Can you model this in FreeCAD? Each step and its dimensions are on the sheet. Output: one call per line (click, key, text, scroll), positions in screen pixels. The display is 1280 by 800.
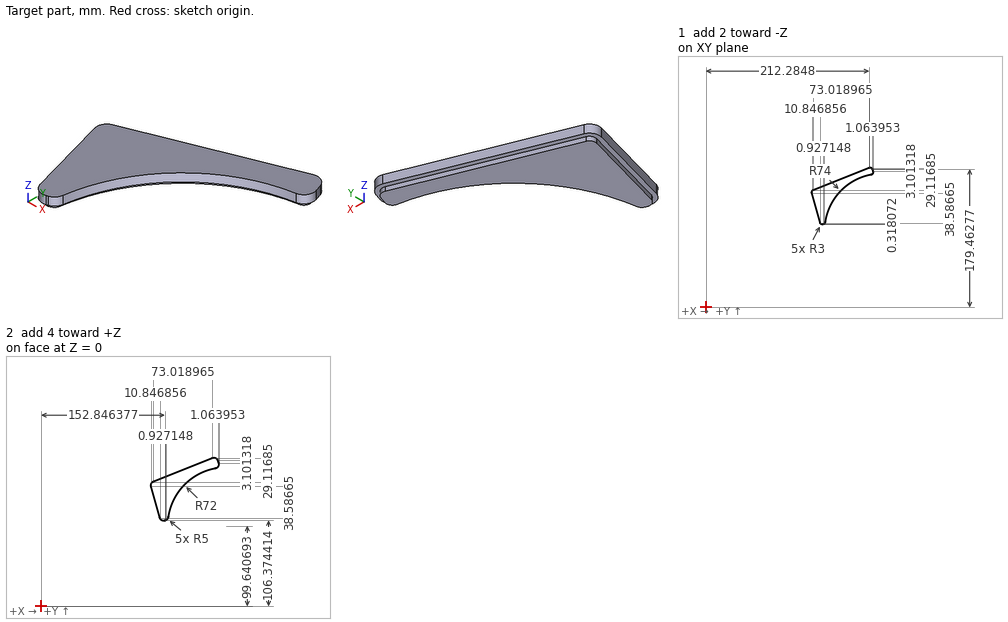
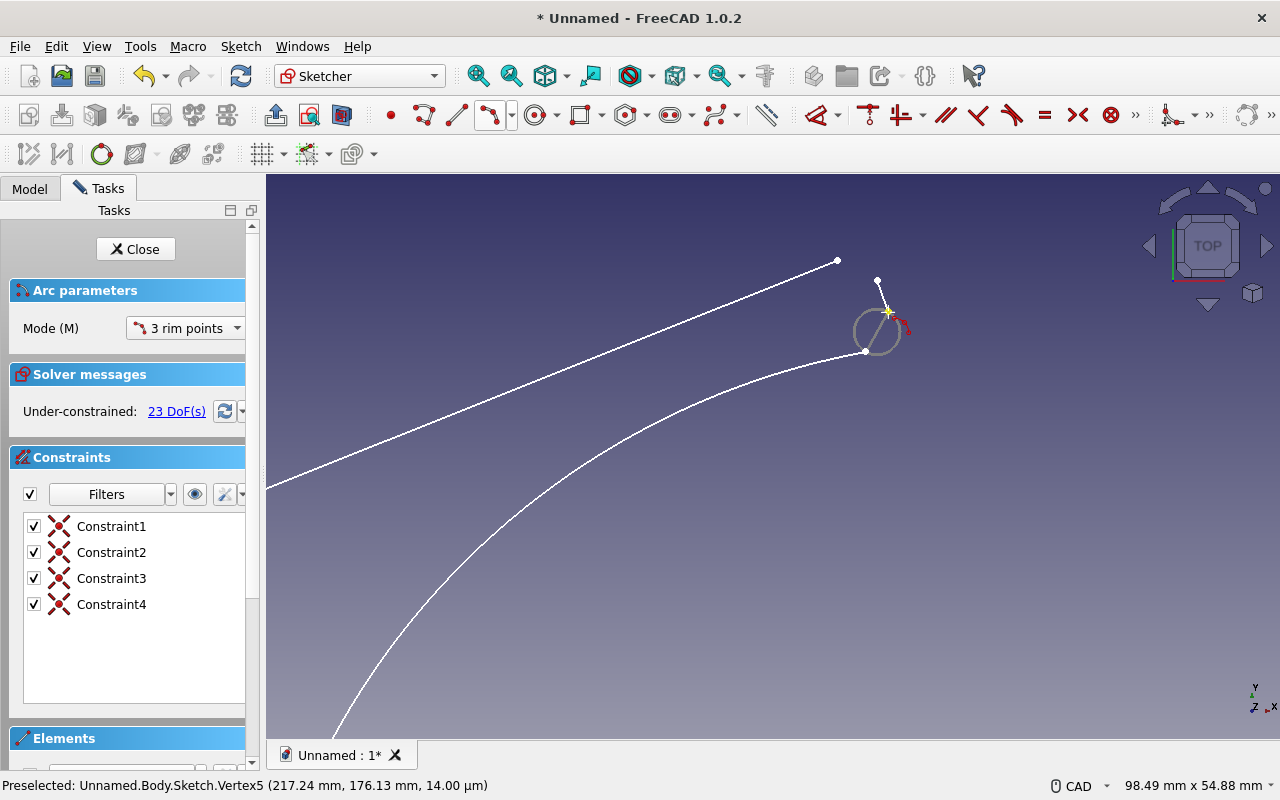
scroll(886, 335, up, 2)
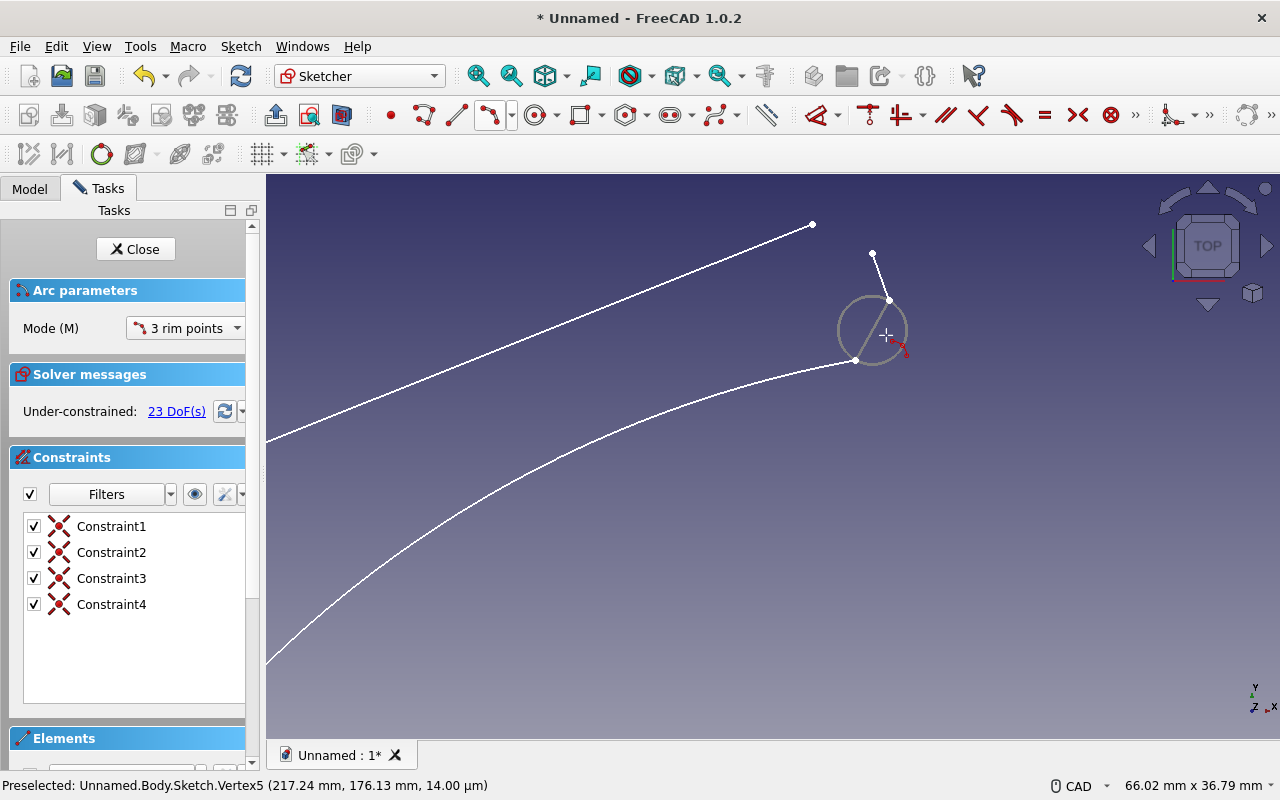
click(886, 335)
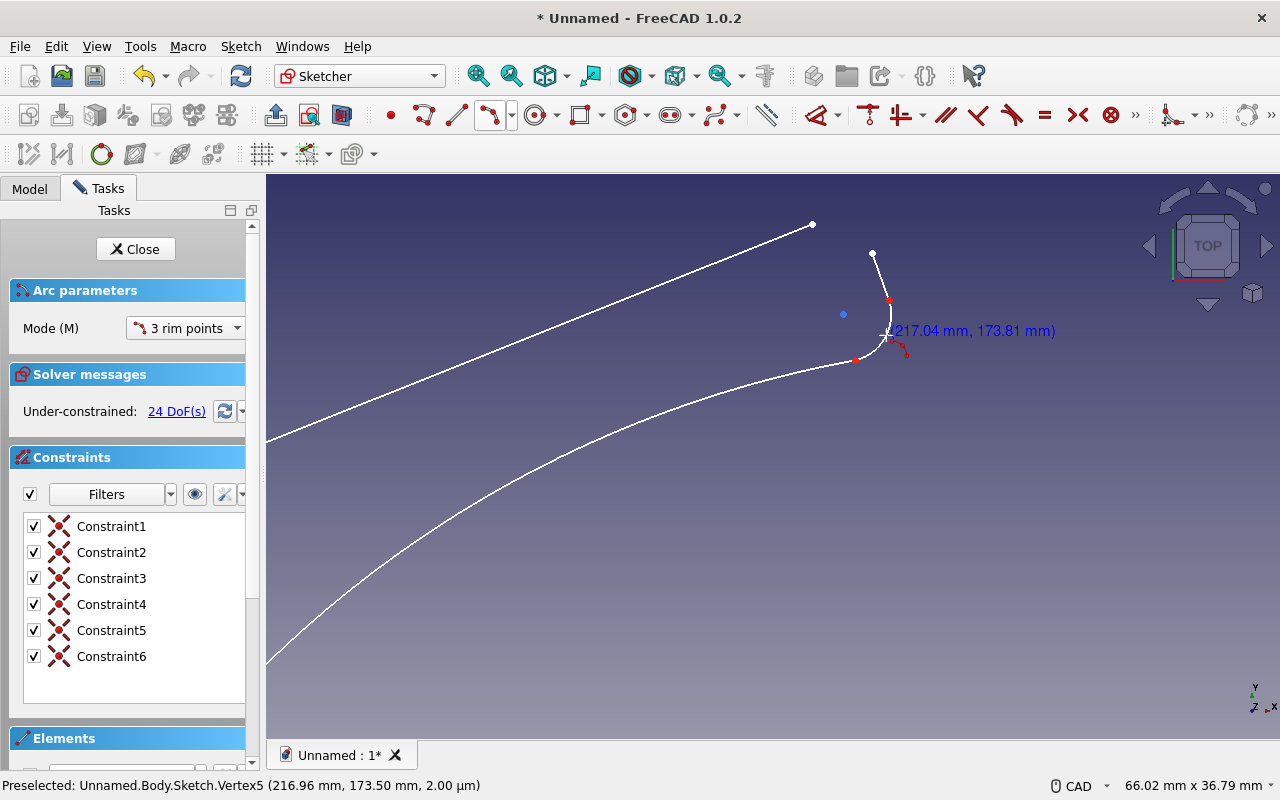
click(872, 254)
click(813, 224)
click(849, 222)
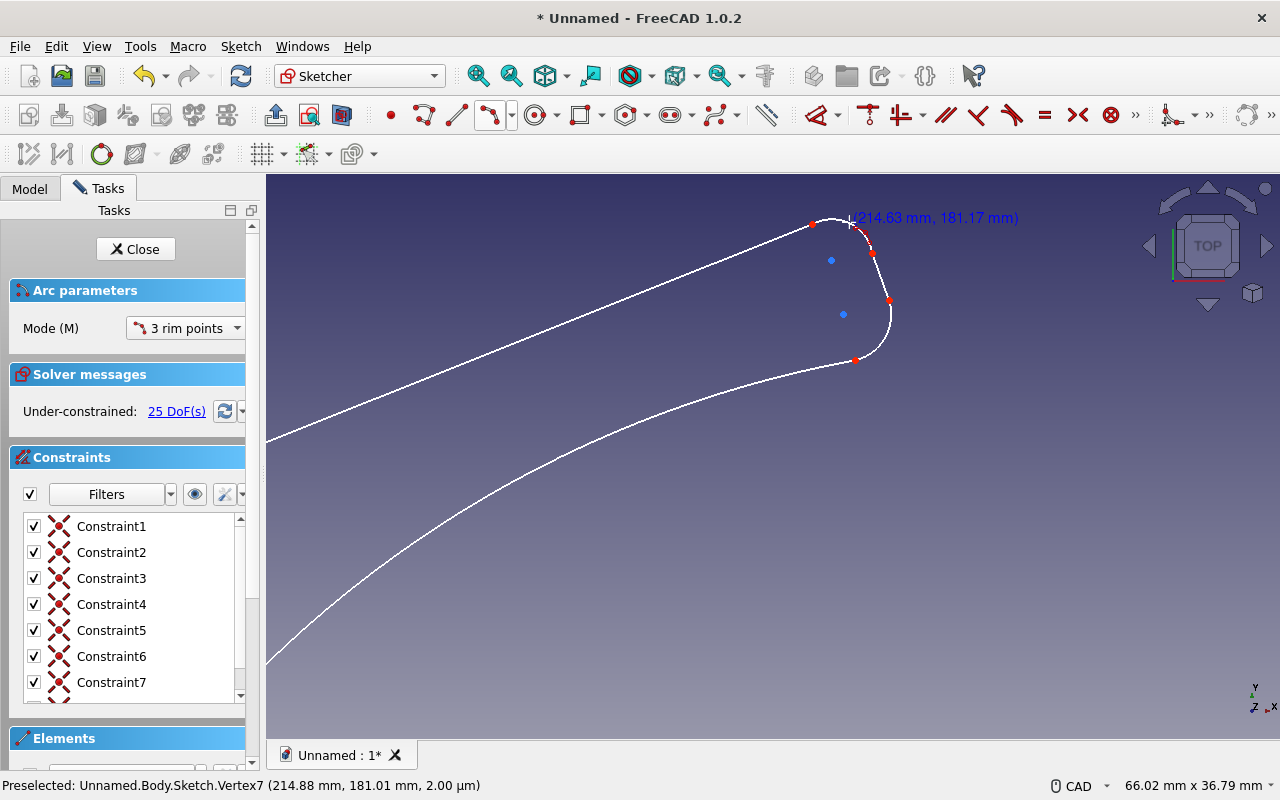
scroll(889, 315, down, 6)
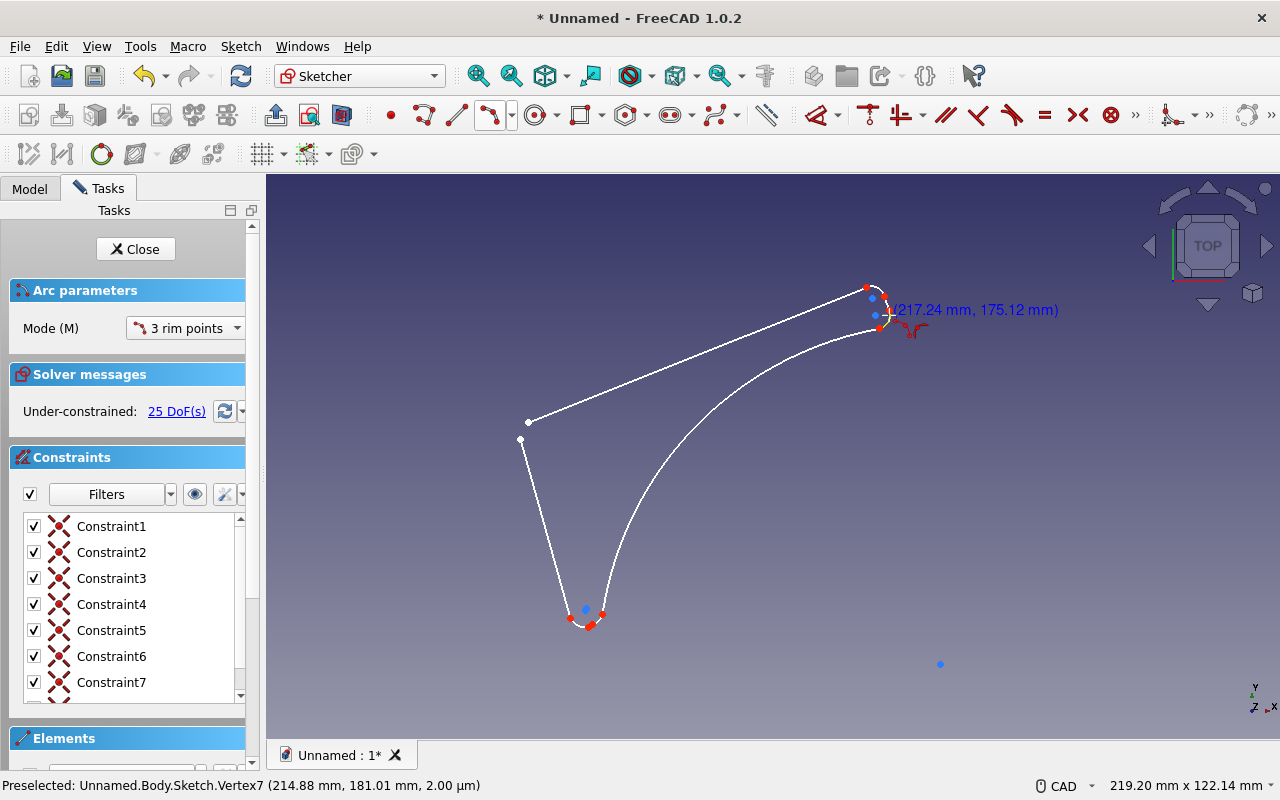
click(528, 423)
click(520, 439)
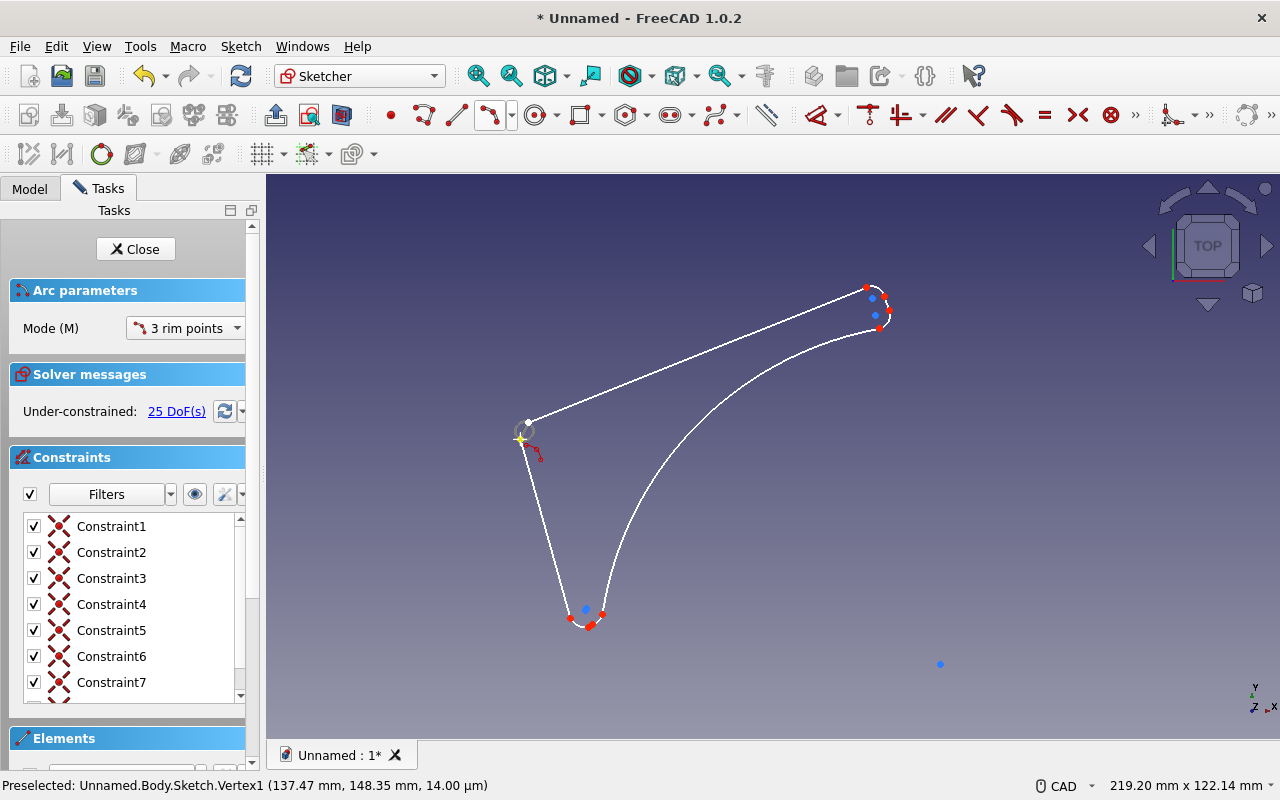
scroll(521, 428, up, 8)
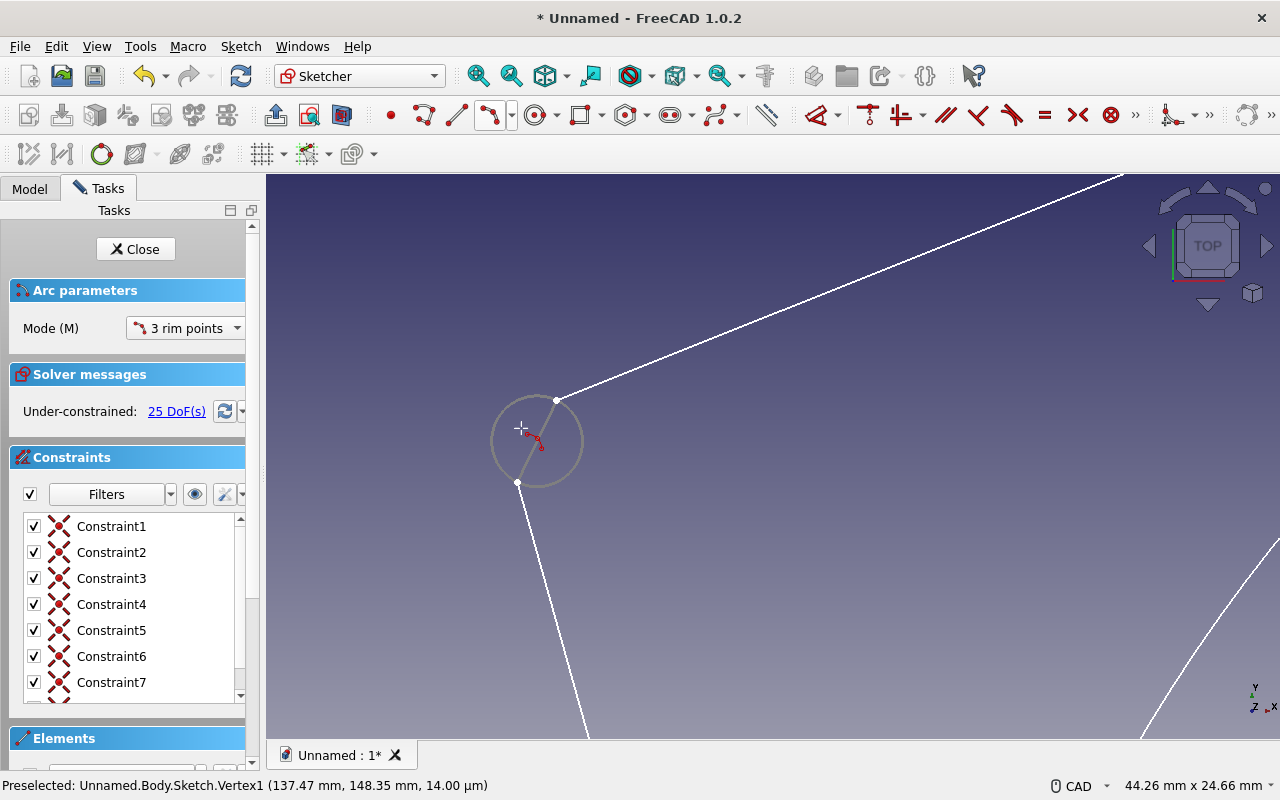
click(522, 428)
key(Escape)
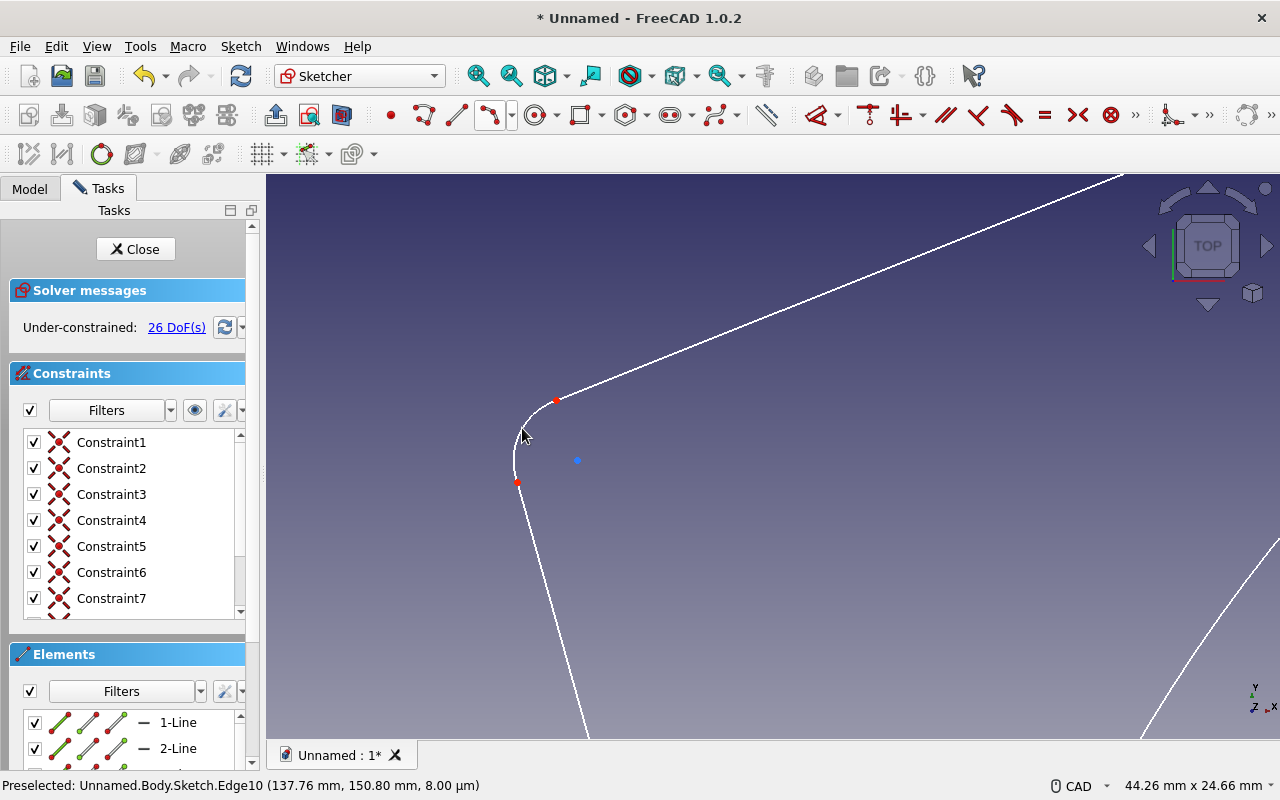
scroll(520, 428, down, 8)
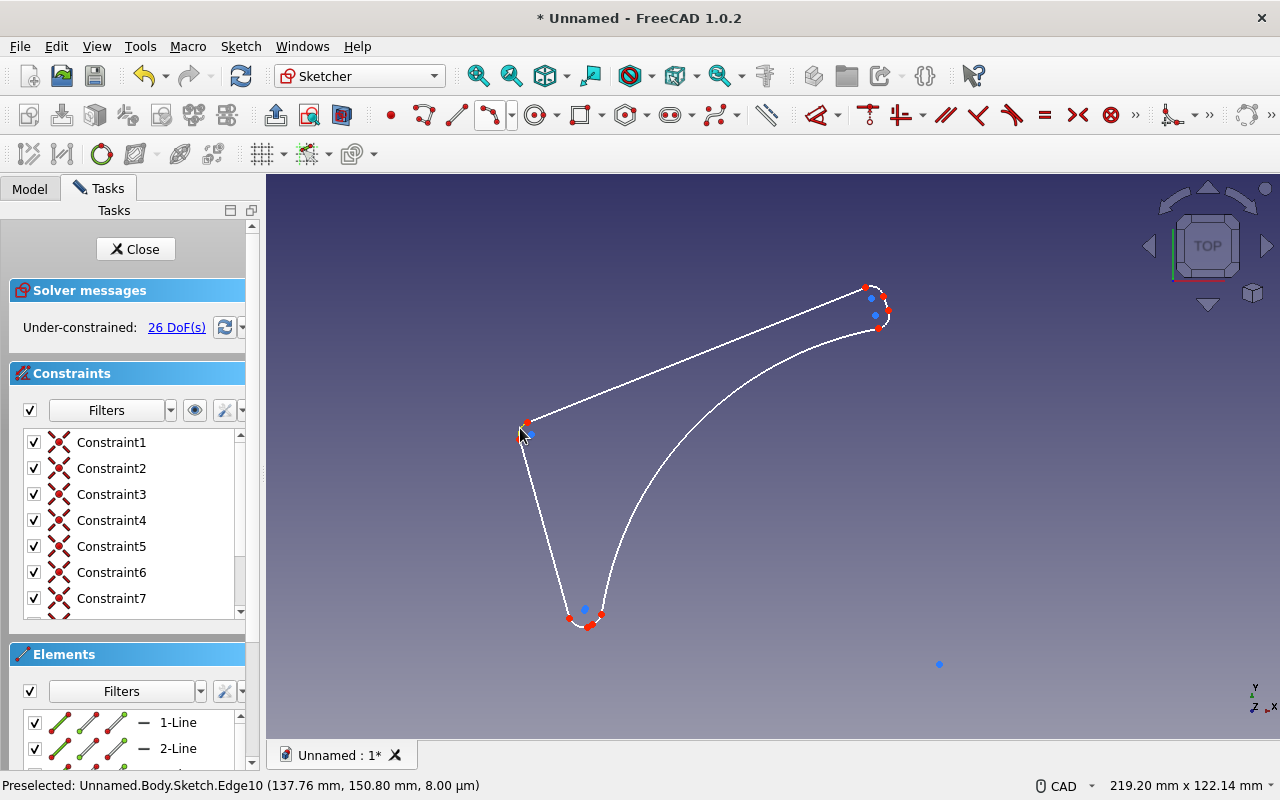
click(530, 475)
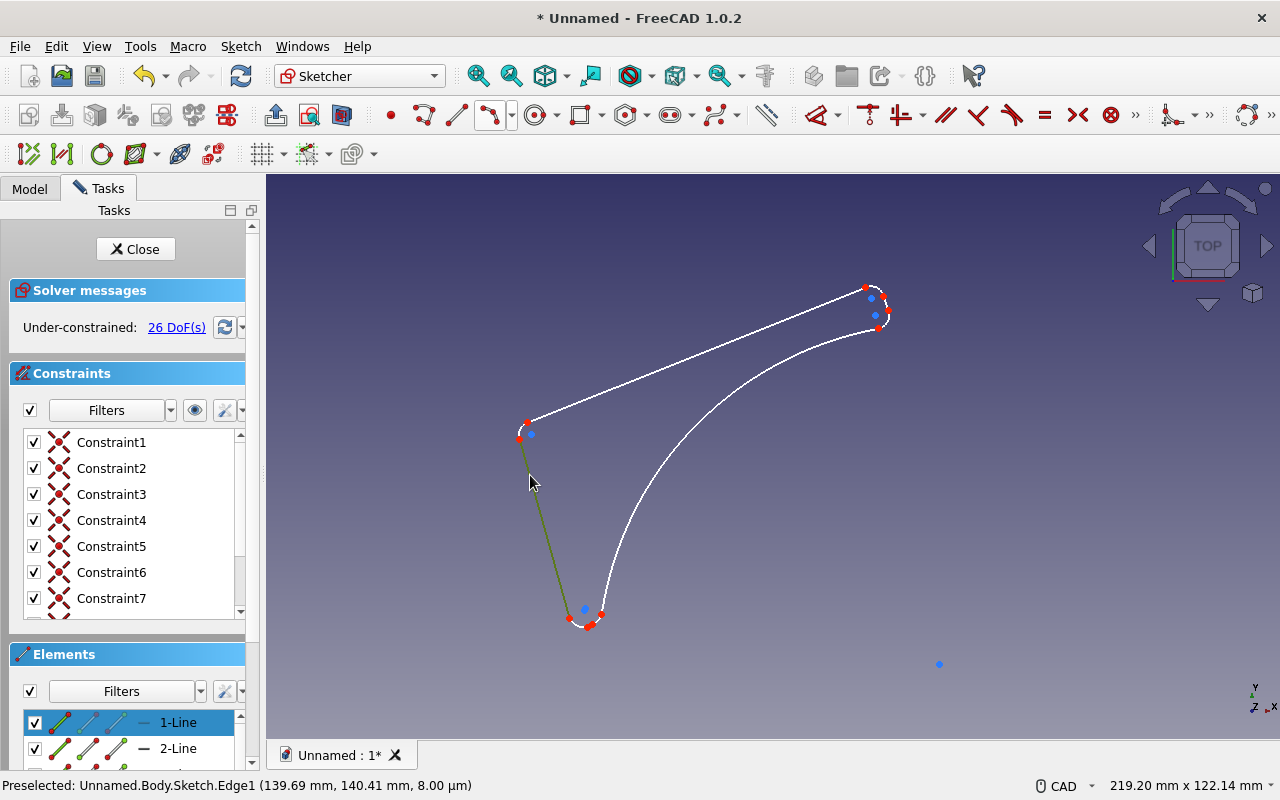
scroll(577, 626, up, 2)